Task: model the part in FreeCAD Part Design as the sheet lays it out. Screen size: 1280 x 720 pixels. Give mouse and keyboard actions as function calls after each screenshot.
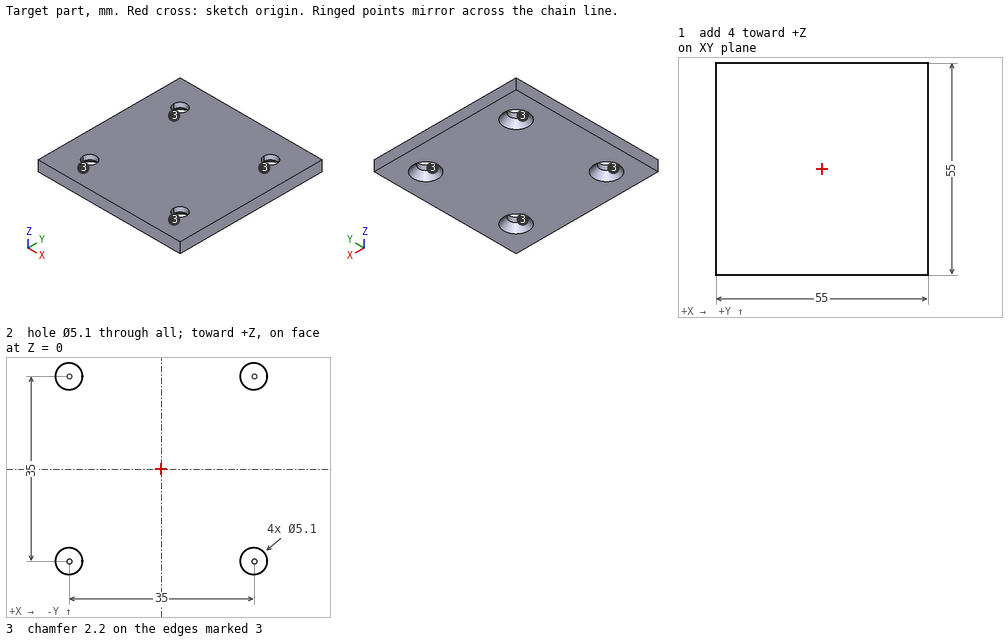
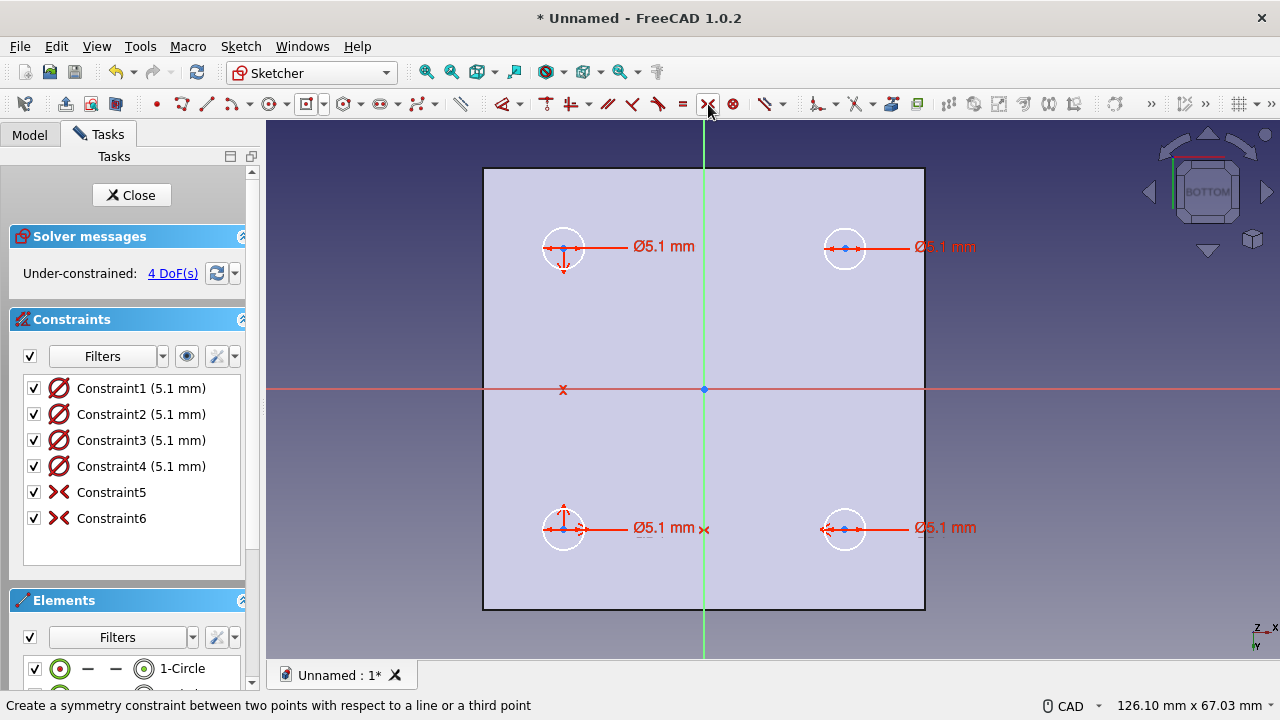
click(845, 530)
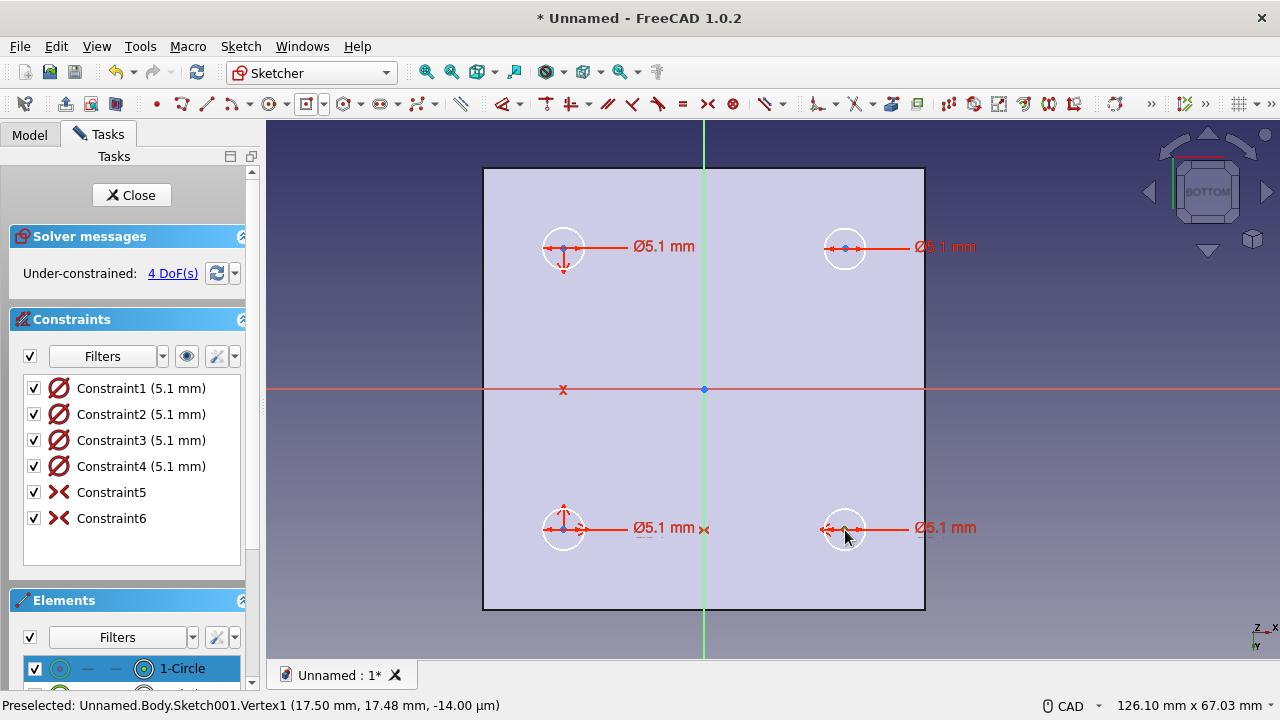
click(845, 249)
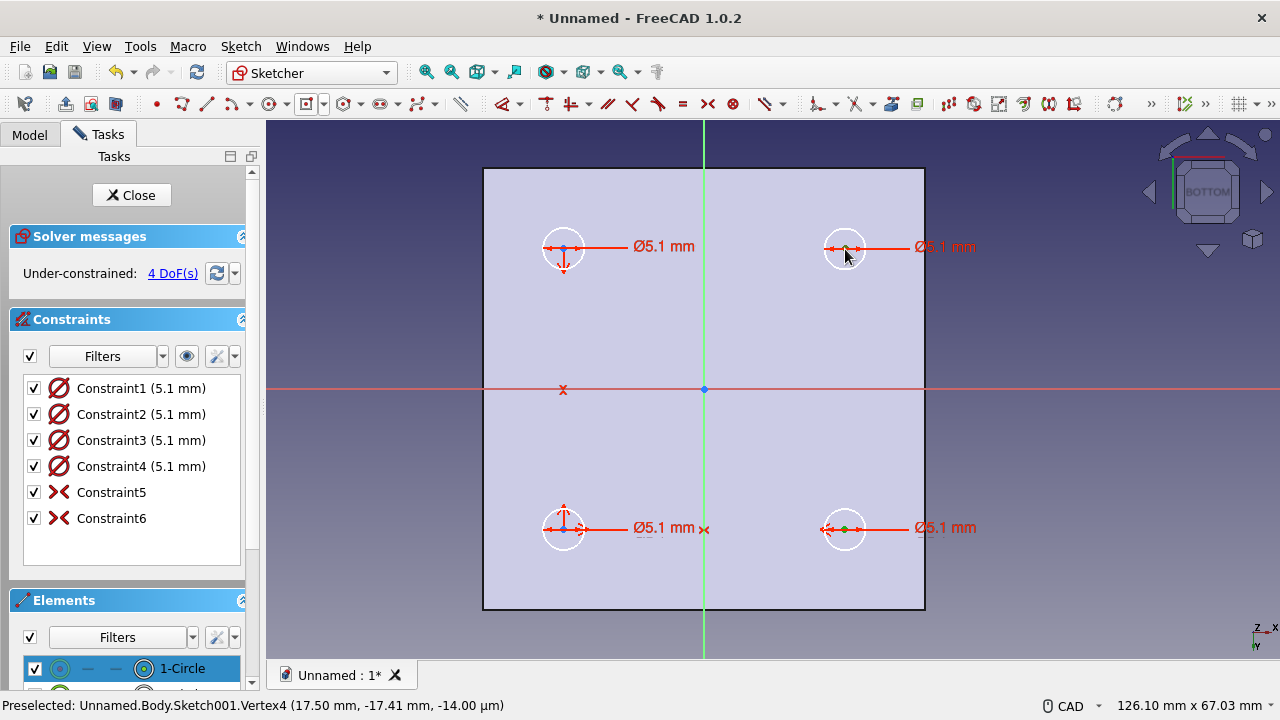
click(353, 389)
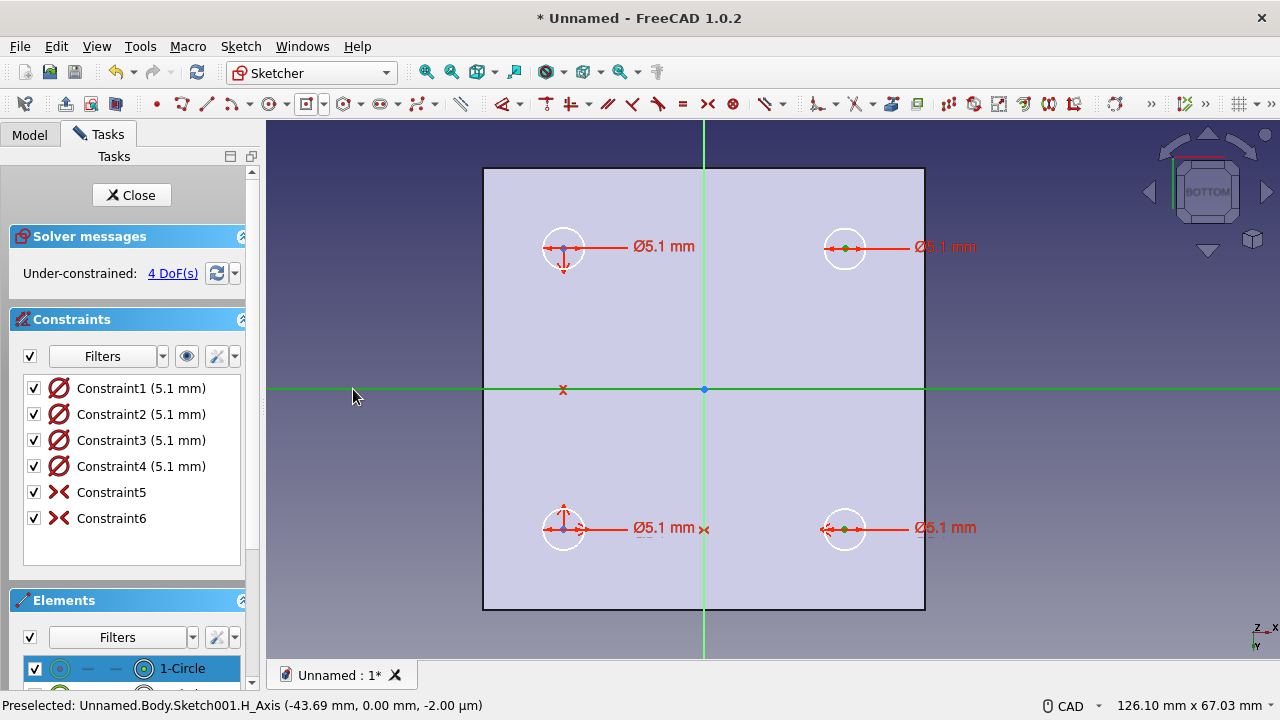
click(708, 104)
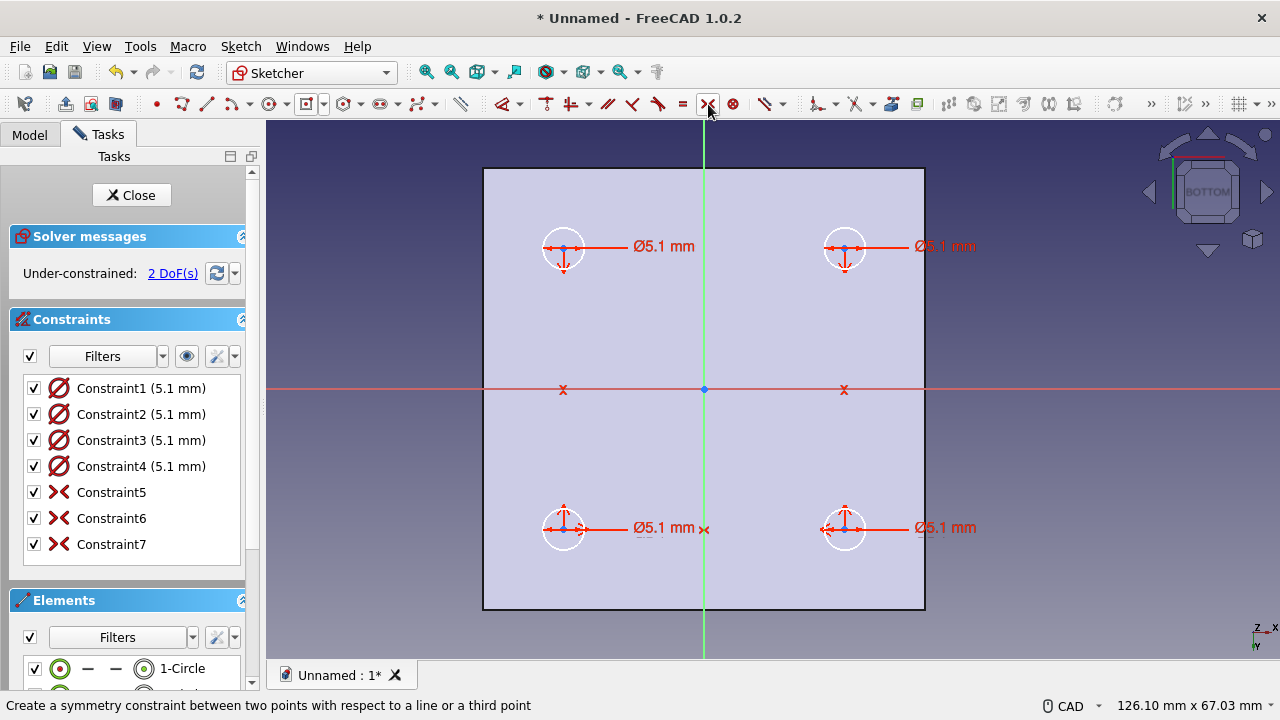
click(502, 104)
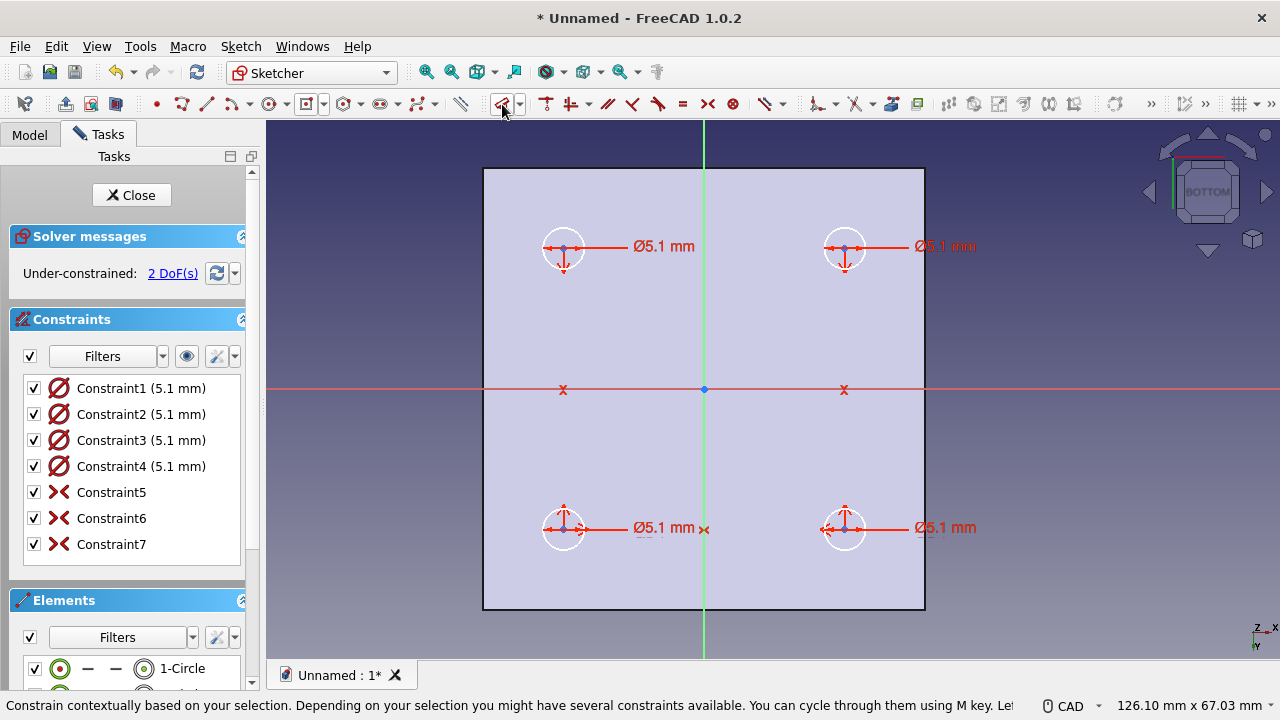
click(845, 530)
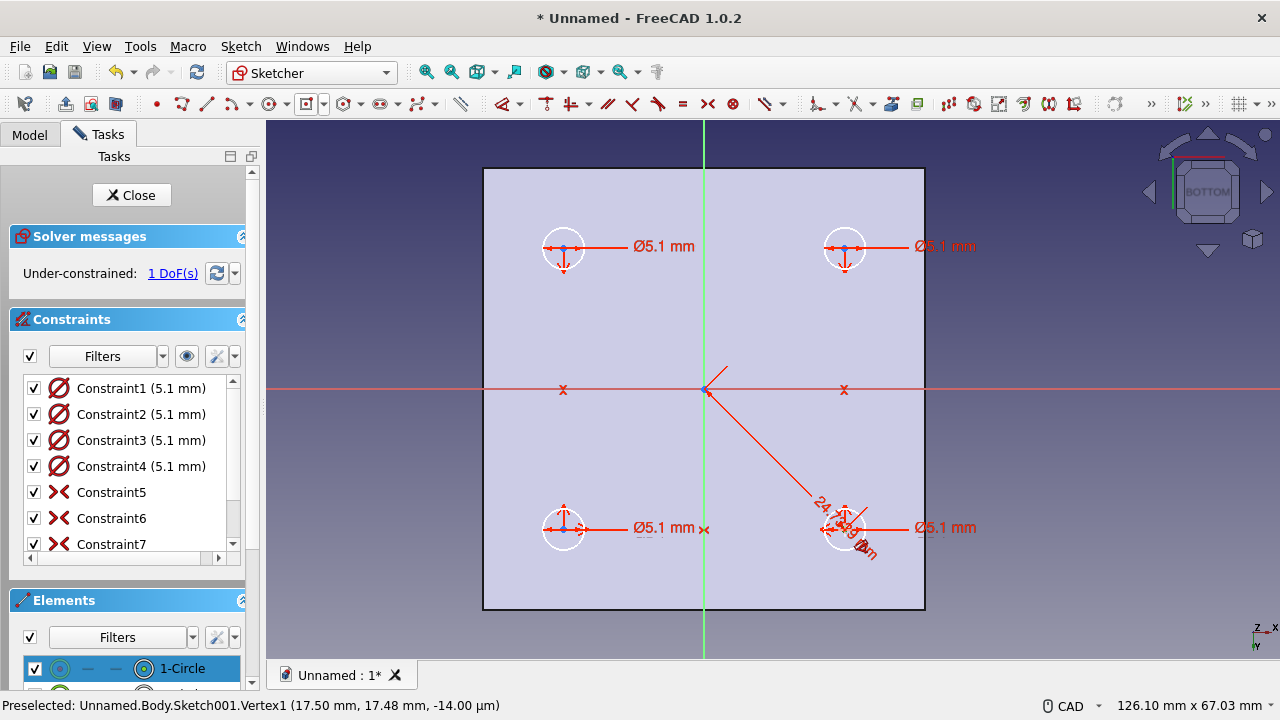
click(564, 530)
click(640, 564)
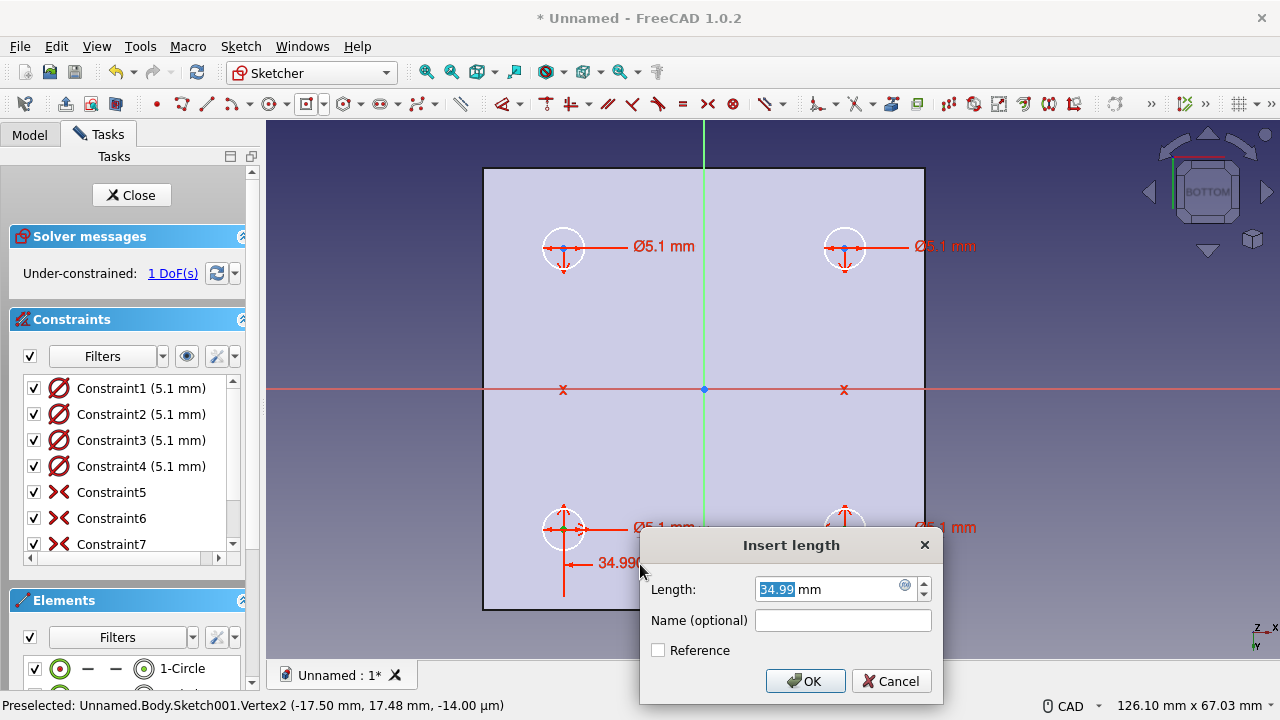
text(35)
key(Return)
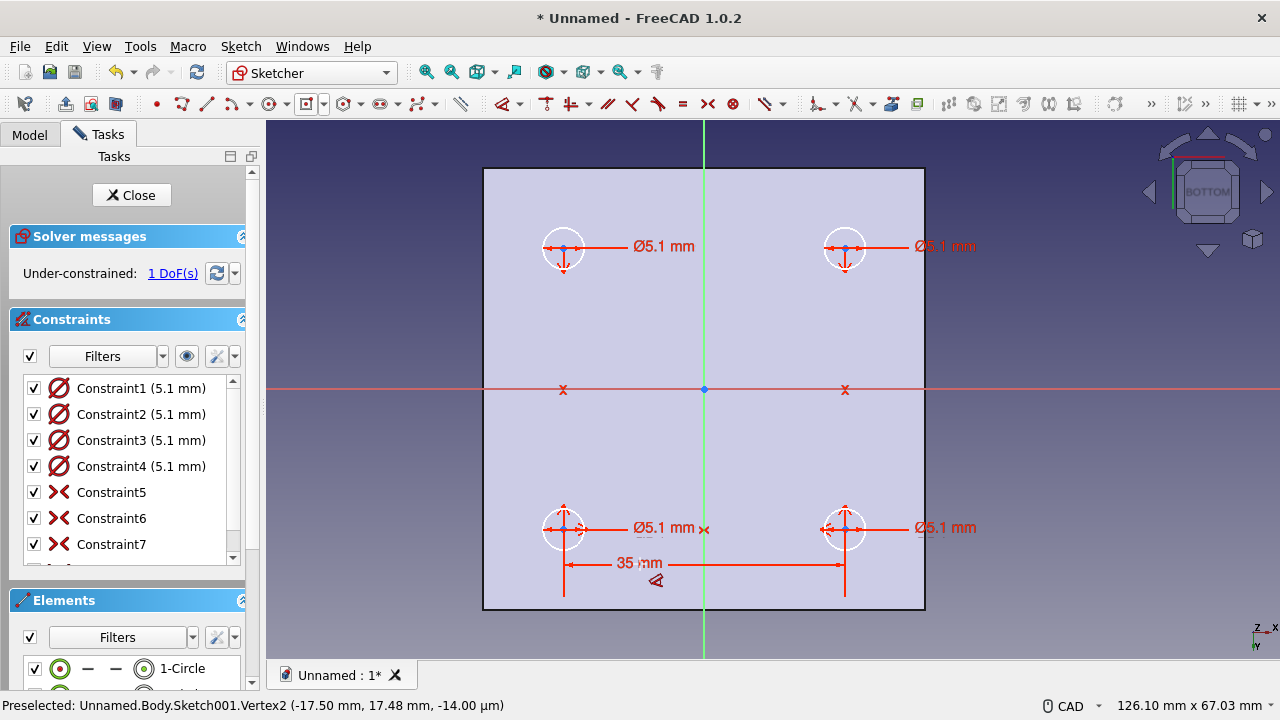
click(564, 530)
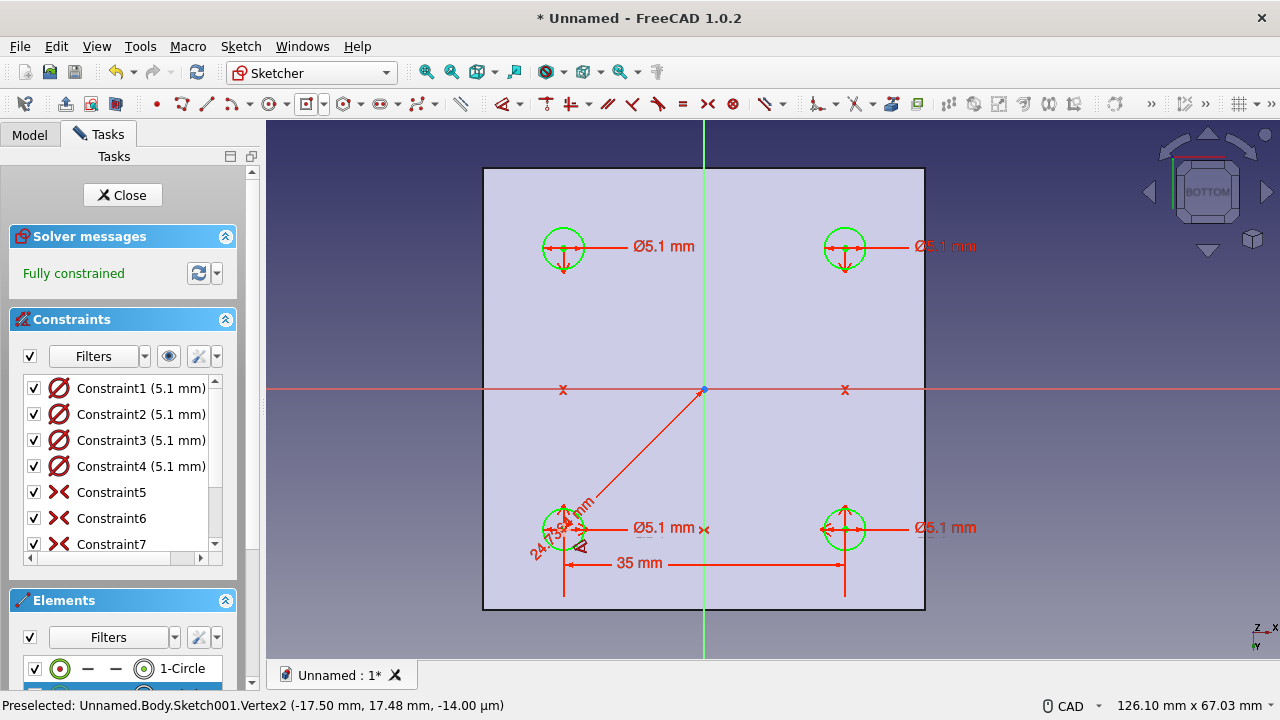
click(564, 248)
click(530, 324)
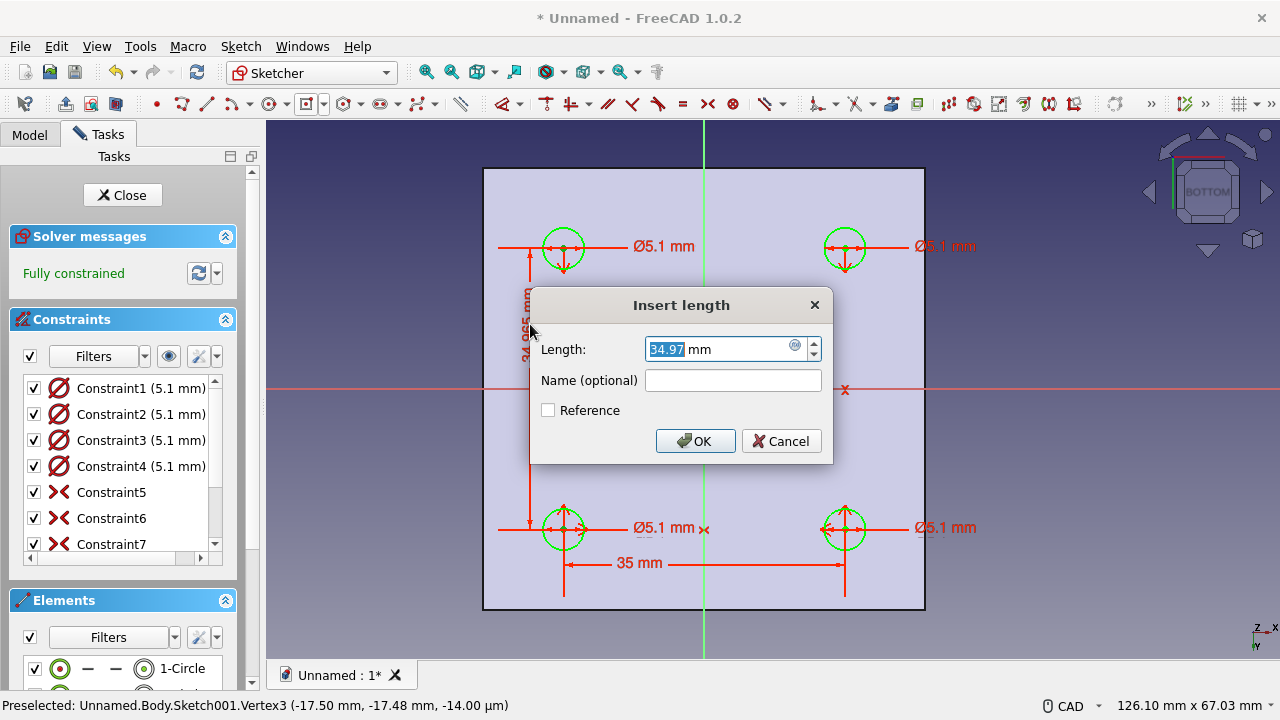
text(35)
key(Return)
key(Escape)